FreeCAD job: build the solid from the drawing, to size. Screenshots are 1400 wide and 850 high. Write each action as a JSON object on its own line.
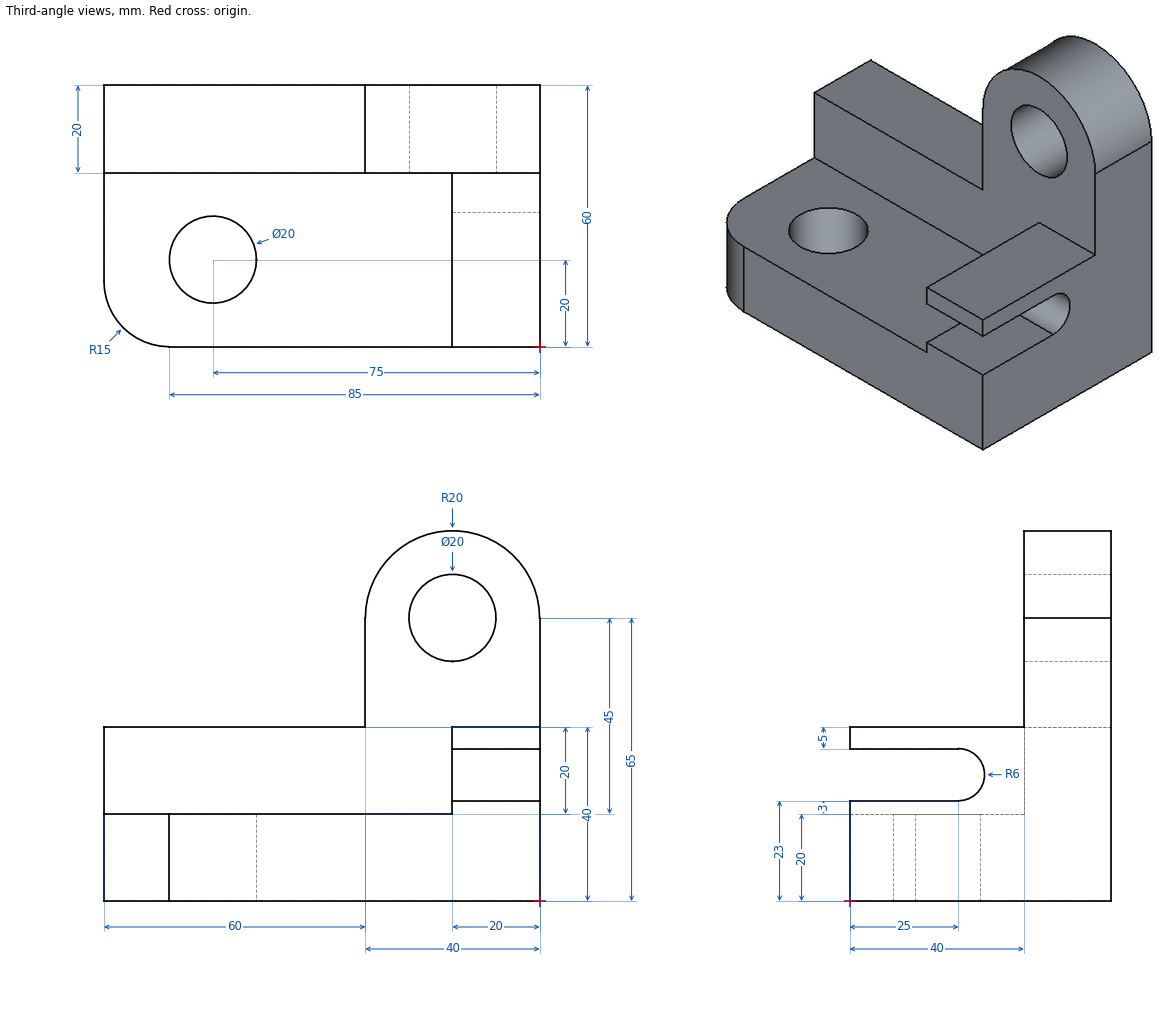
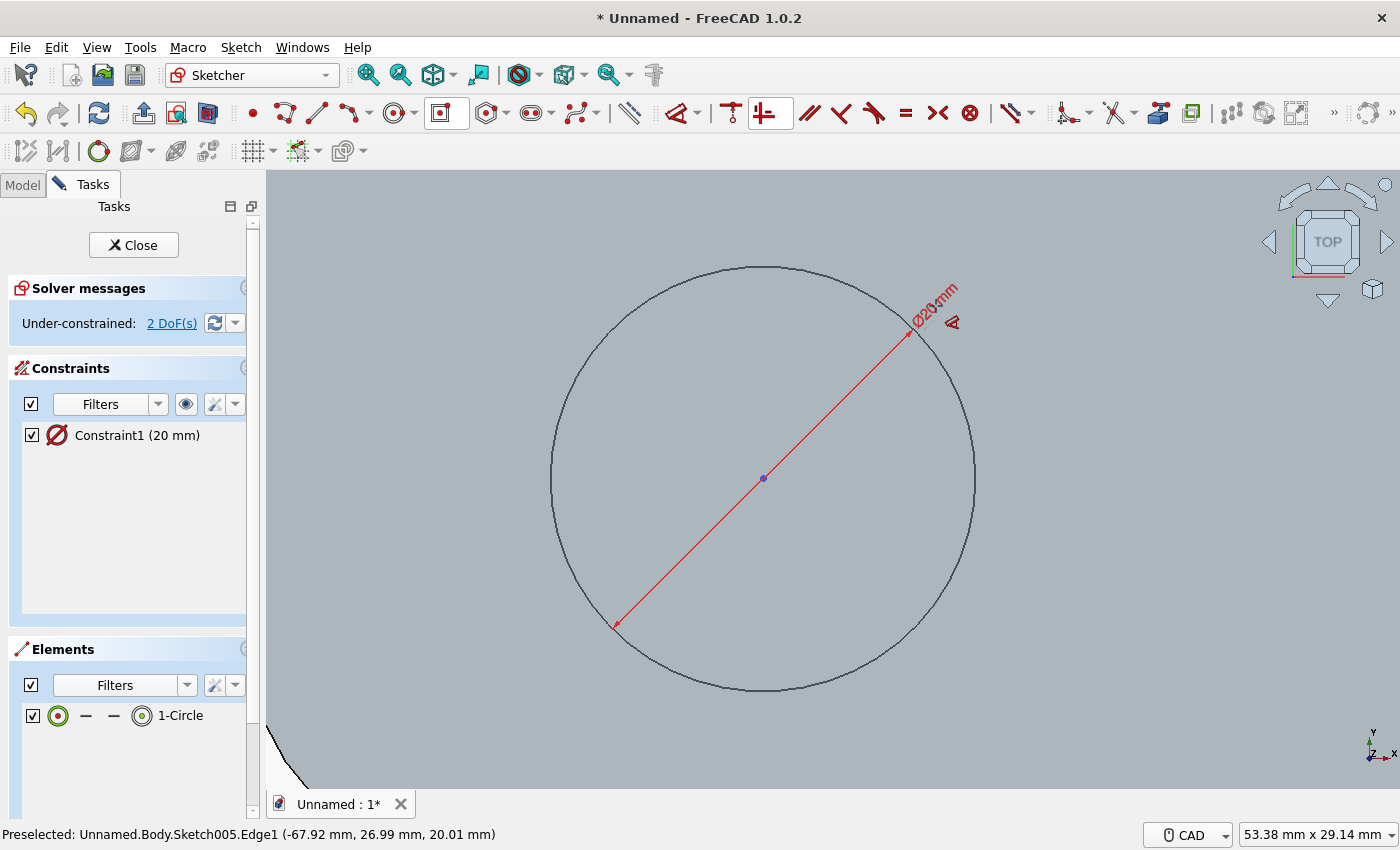
{"action": "left_click", "coordinate": [763, 479]}
{"action": "left_click", "coordinate": [999, 445]}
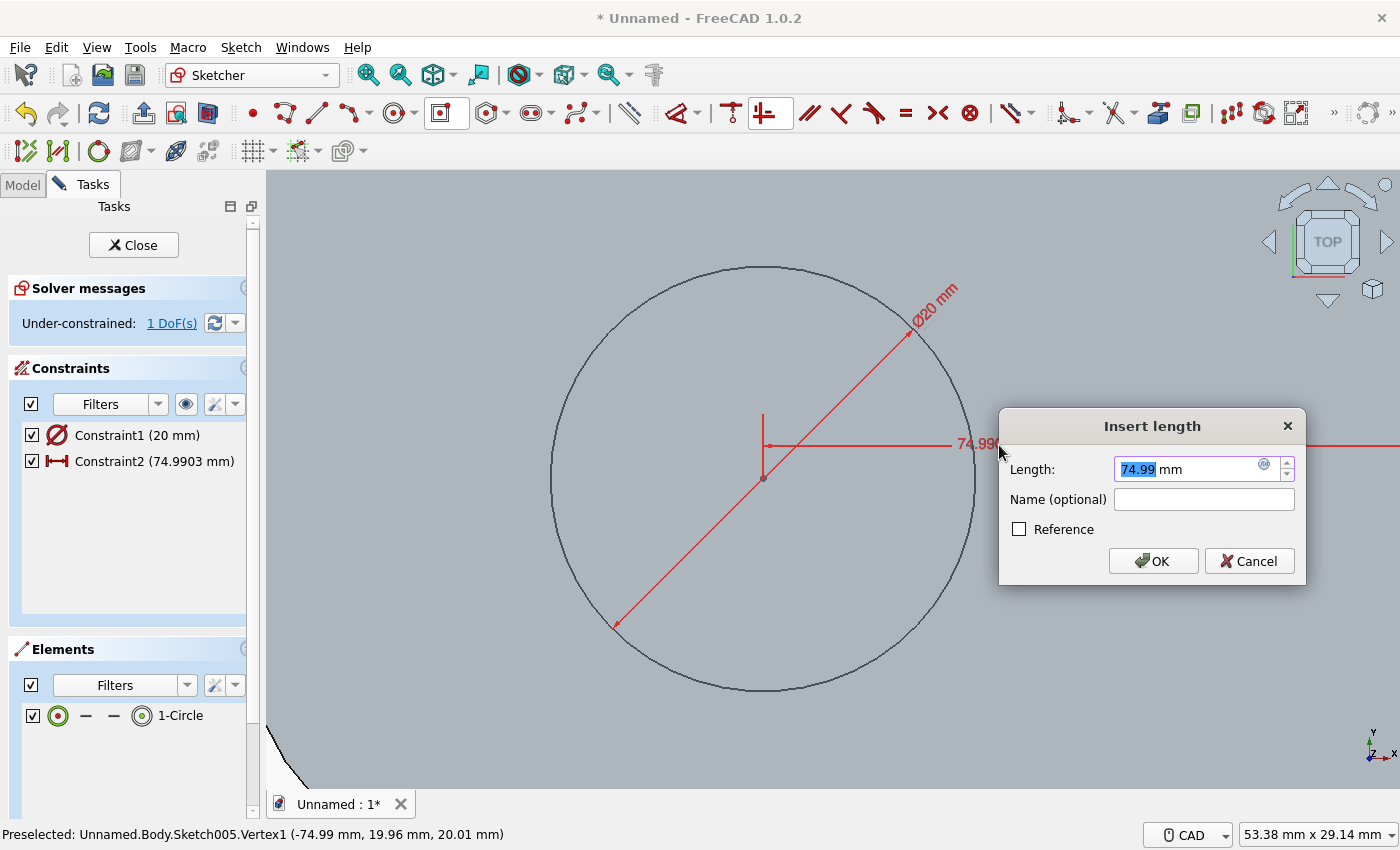
{"action": "type", "text": "75"}
{"action": "key", "text": "Return"}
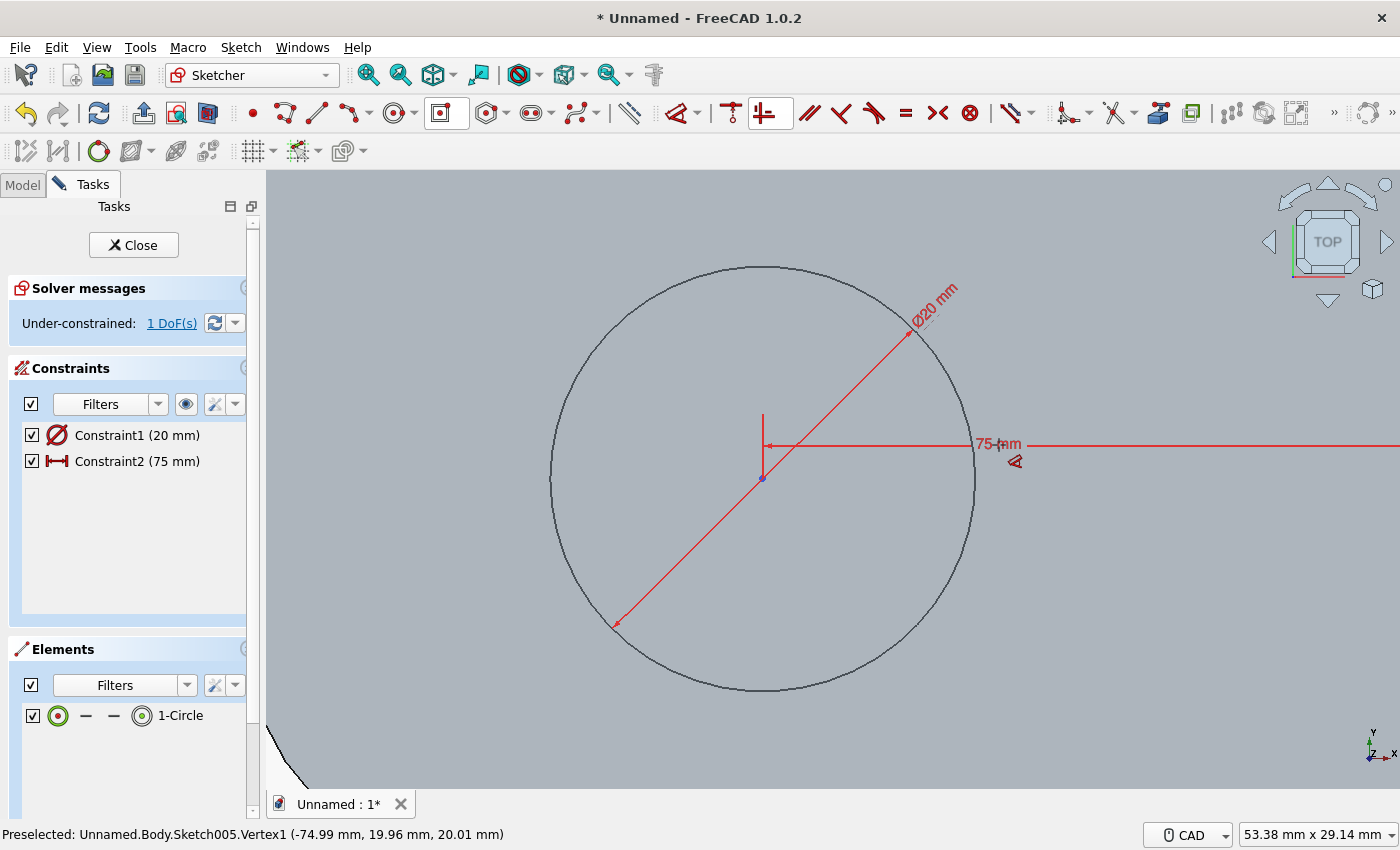
{"action": "left_click", "coordinate": [763, 479]}
{"action": "left_click", "coordinate": [729, 620]}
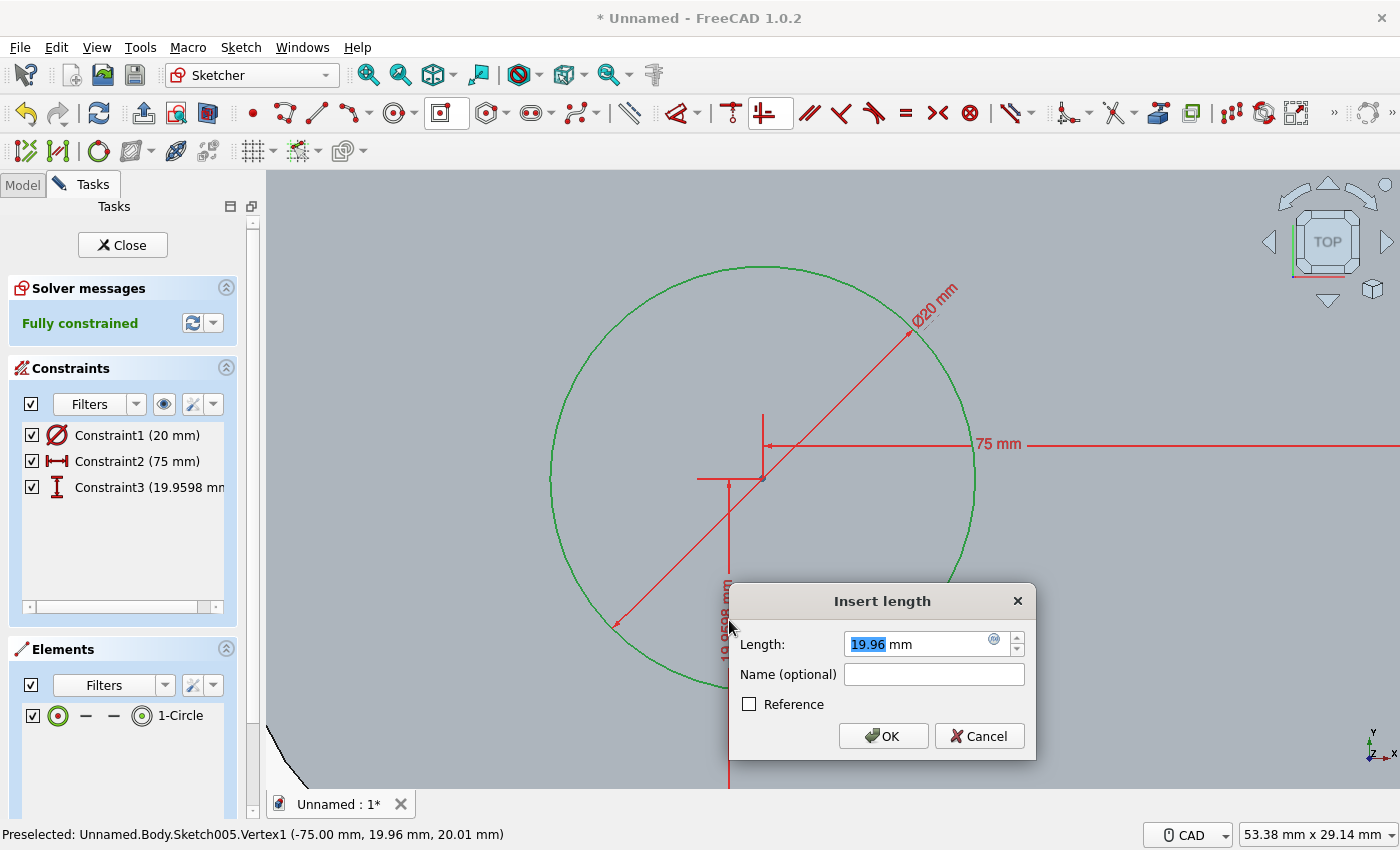
{"action": "type", "text": "20"}
{"action": "key", "text": "Return"}
{"action": "key", "text": "Escape"}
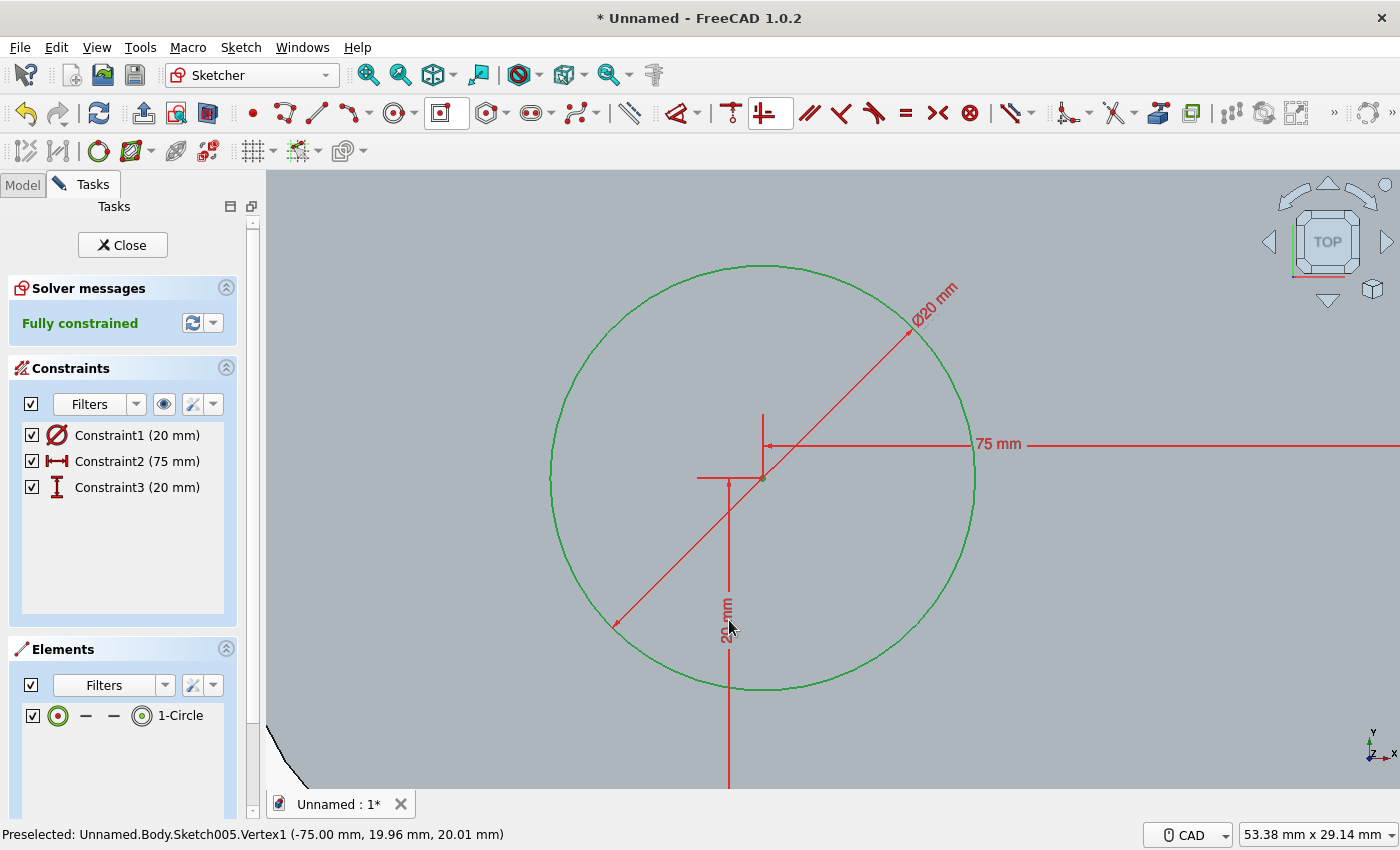
{"action": "left_click", "coordinate": [123, 245]}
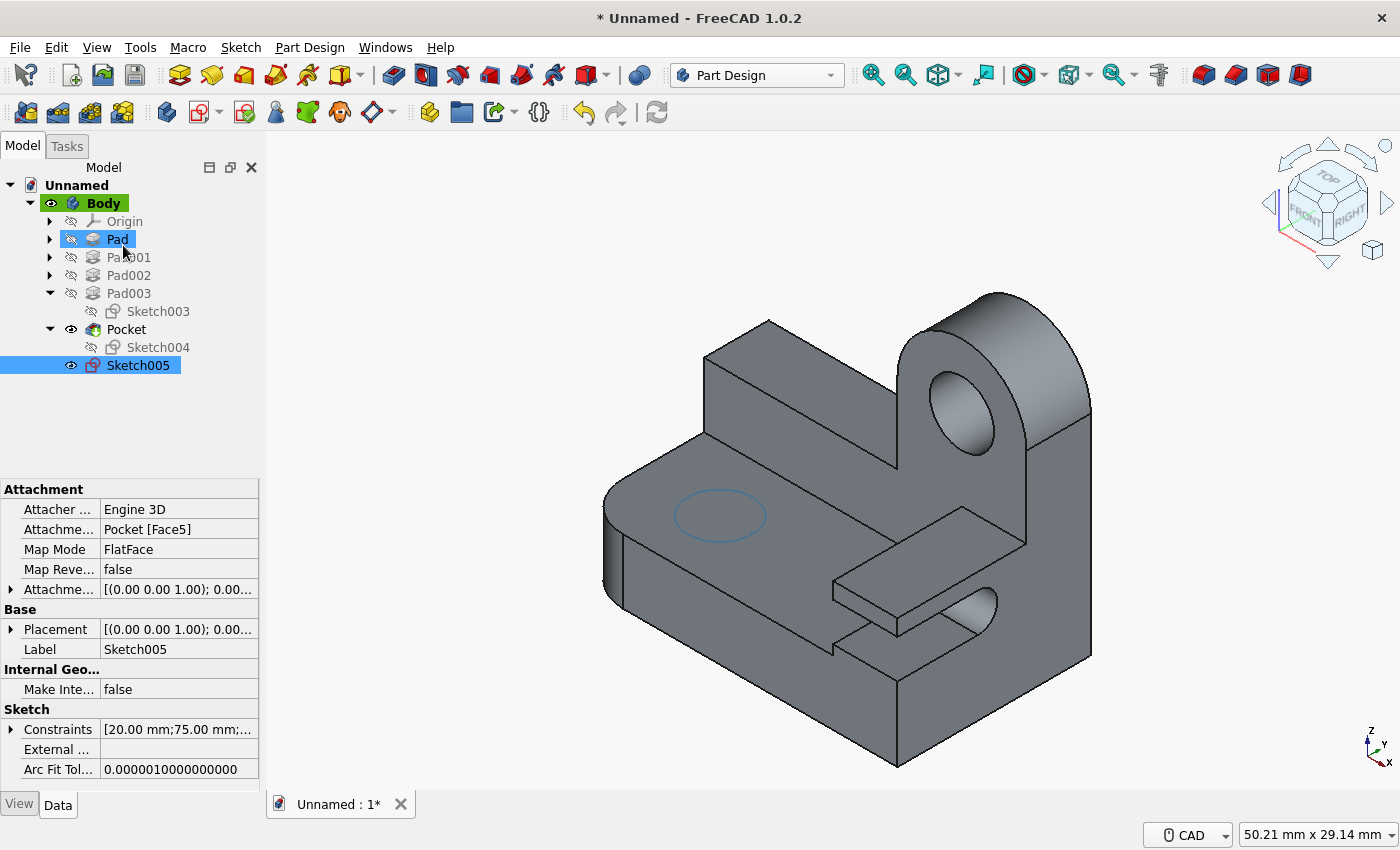
{"action": "left_click", "coordinate": [394, 76]}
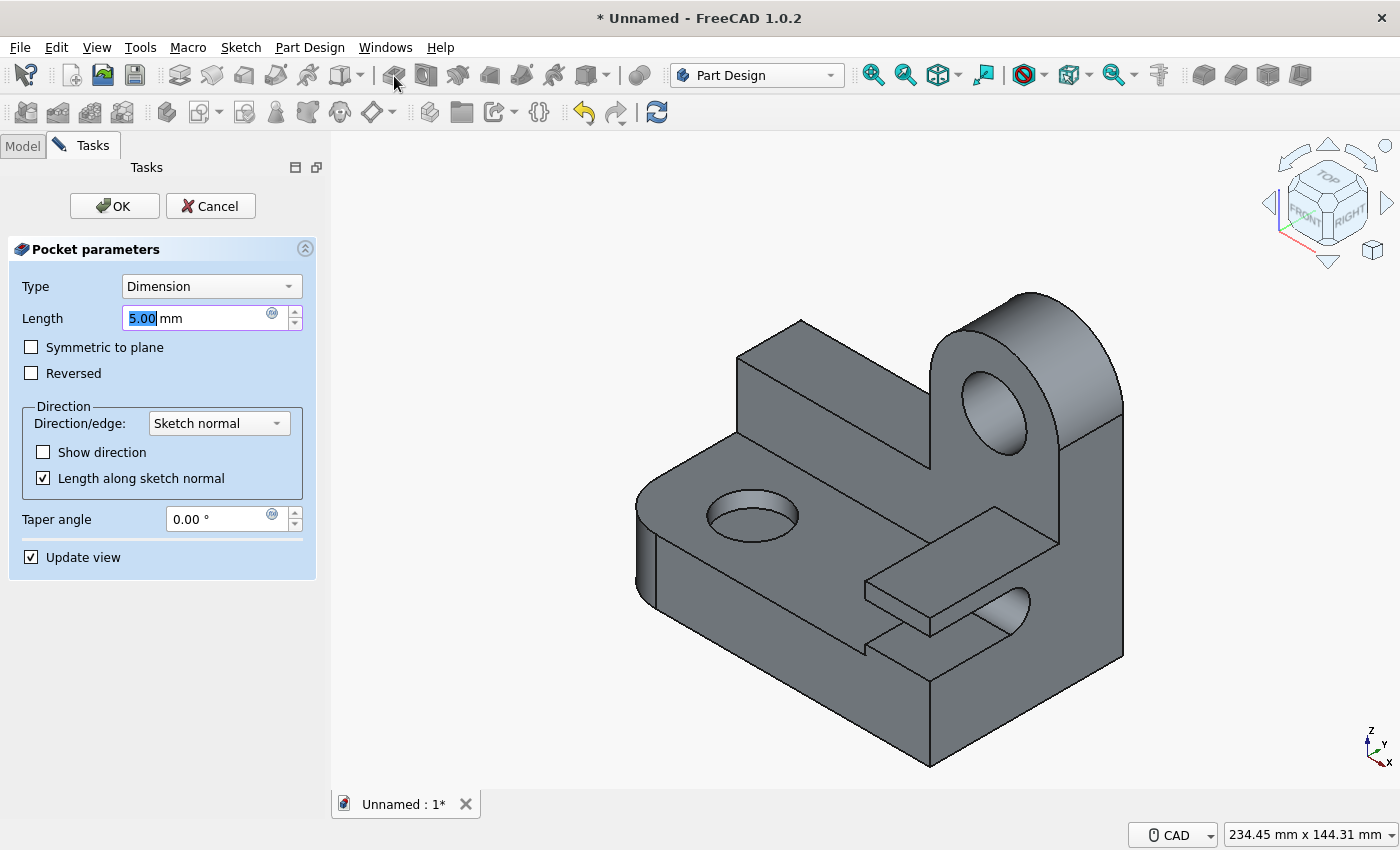
{"action": "type", "text": "20"}
{"action": "key", "text": "Tab"}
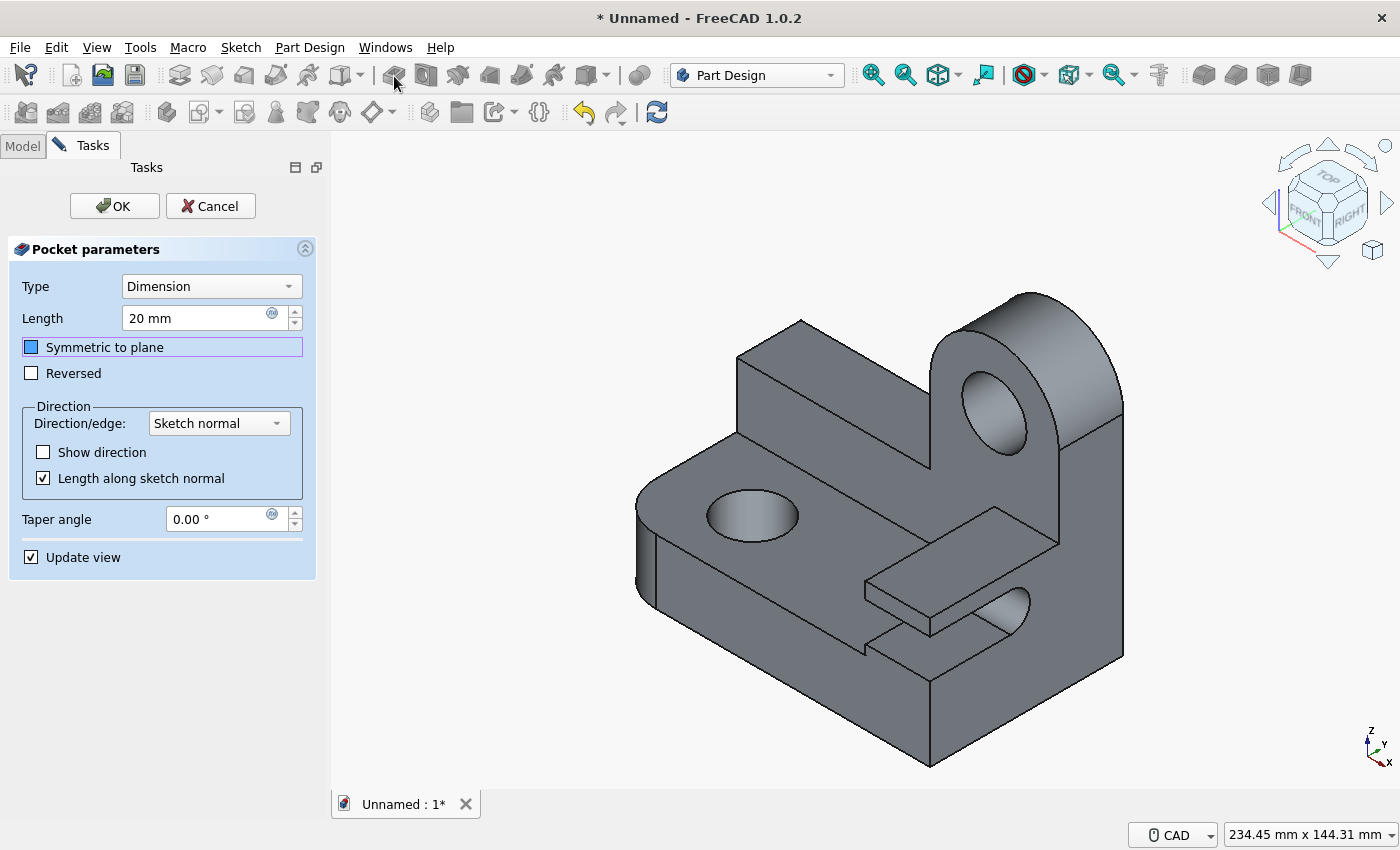
{"action": "left_click", "coordinate": [115, 206]}